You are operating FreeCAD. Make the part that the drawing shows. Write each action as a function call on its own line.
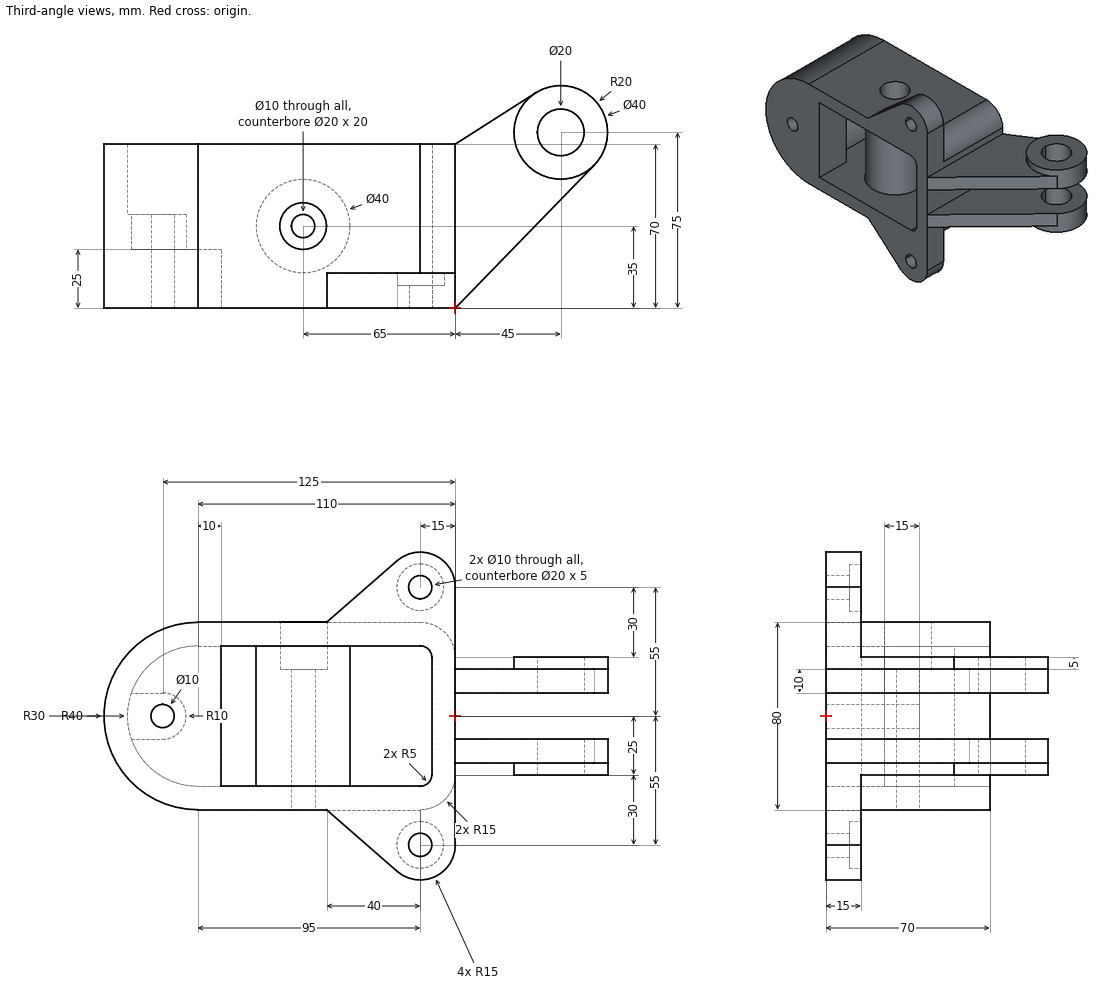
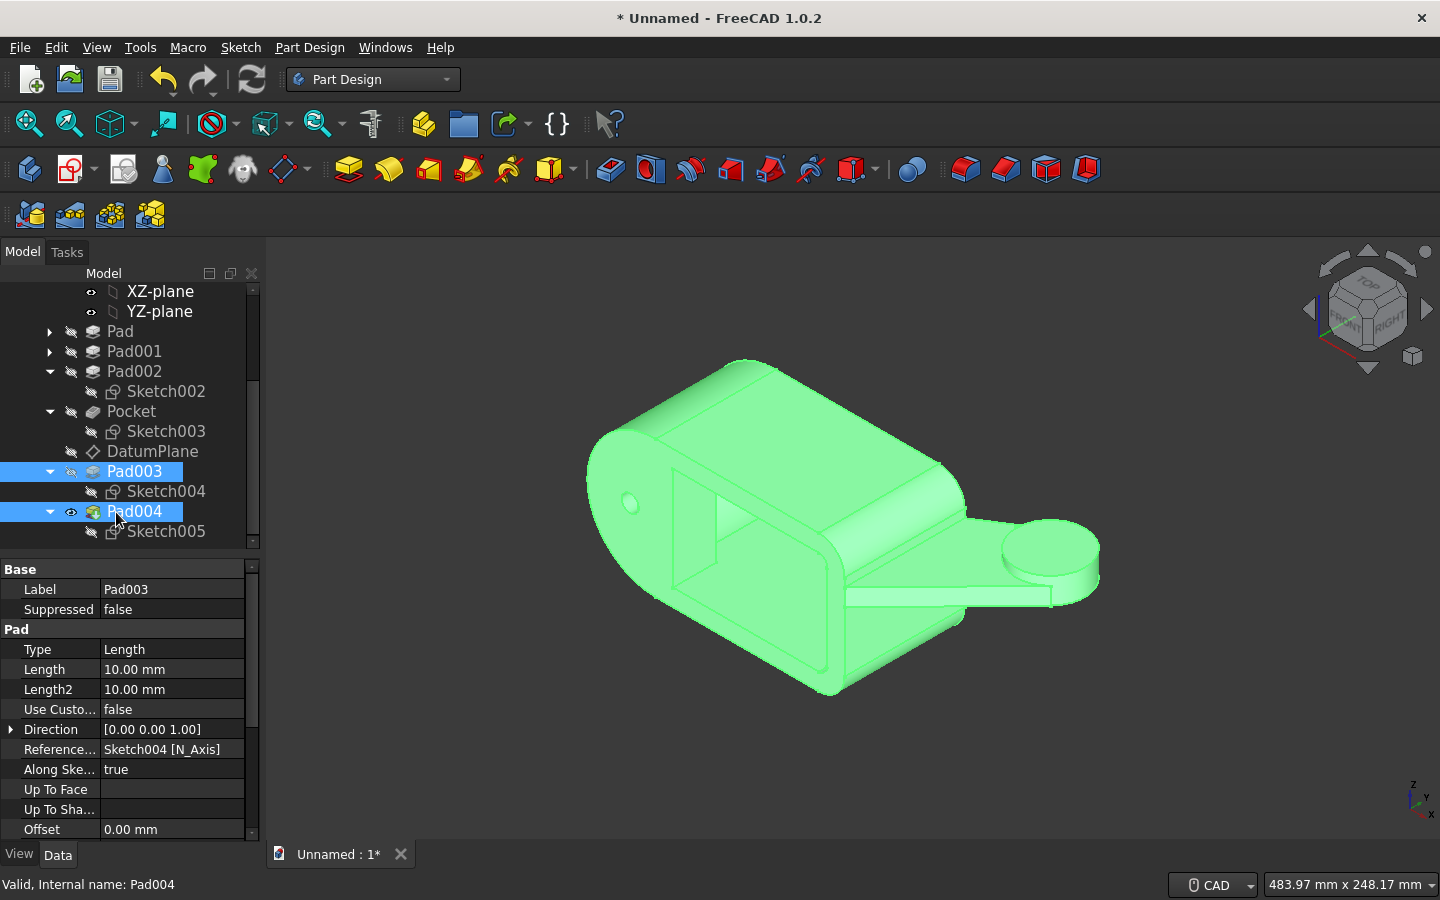
click(30, 214)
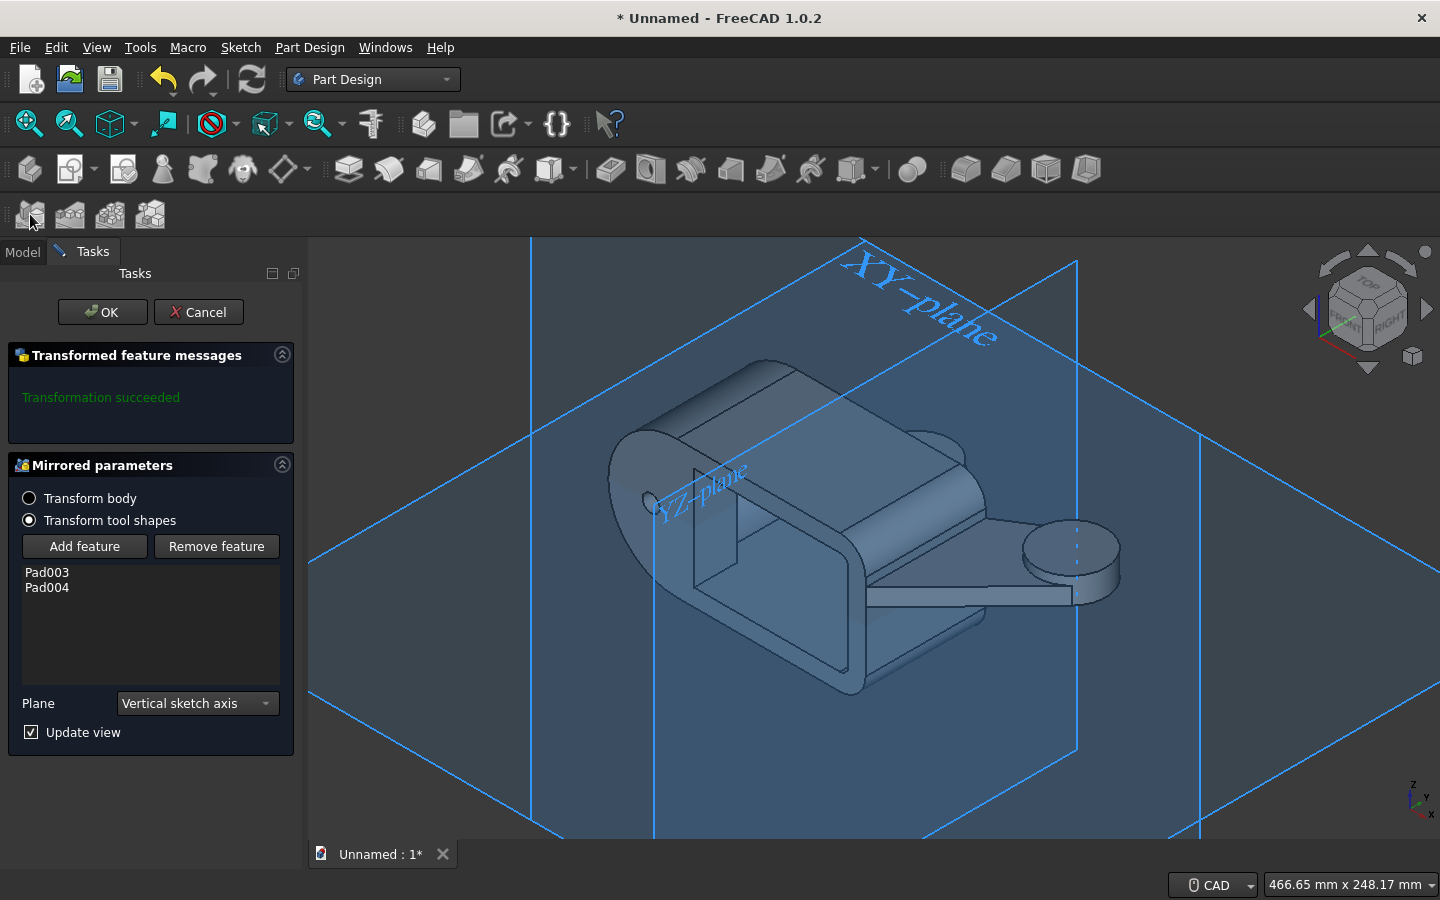
click(198, 704)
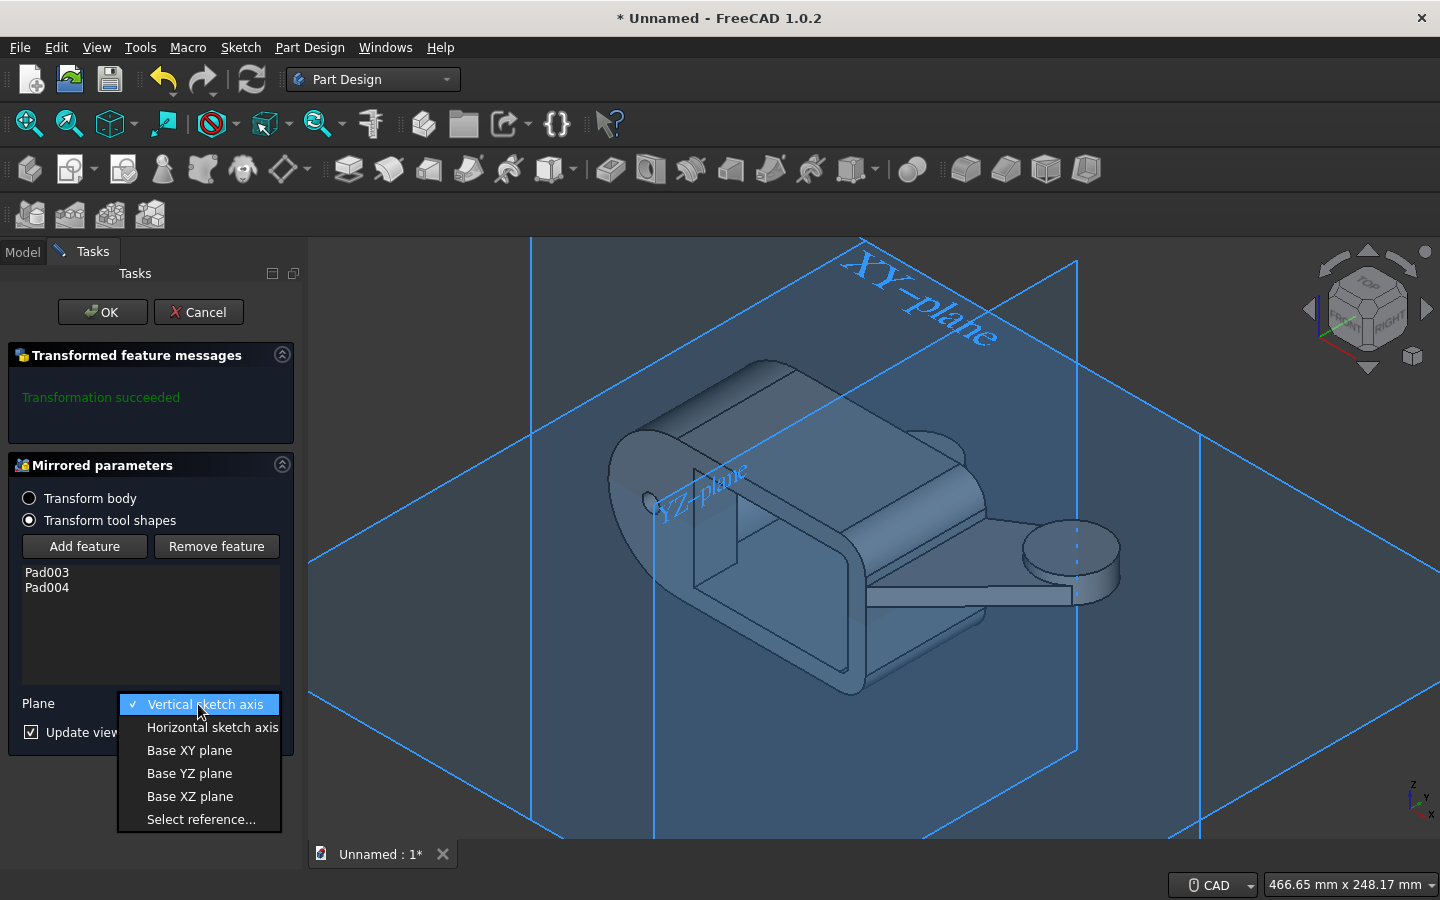
click(198, 750)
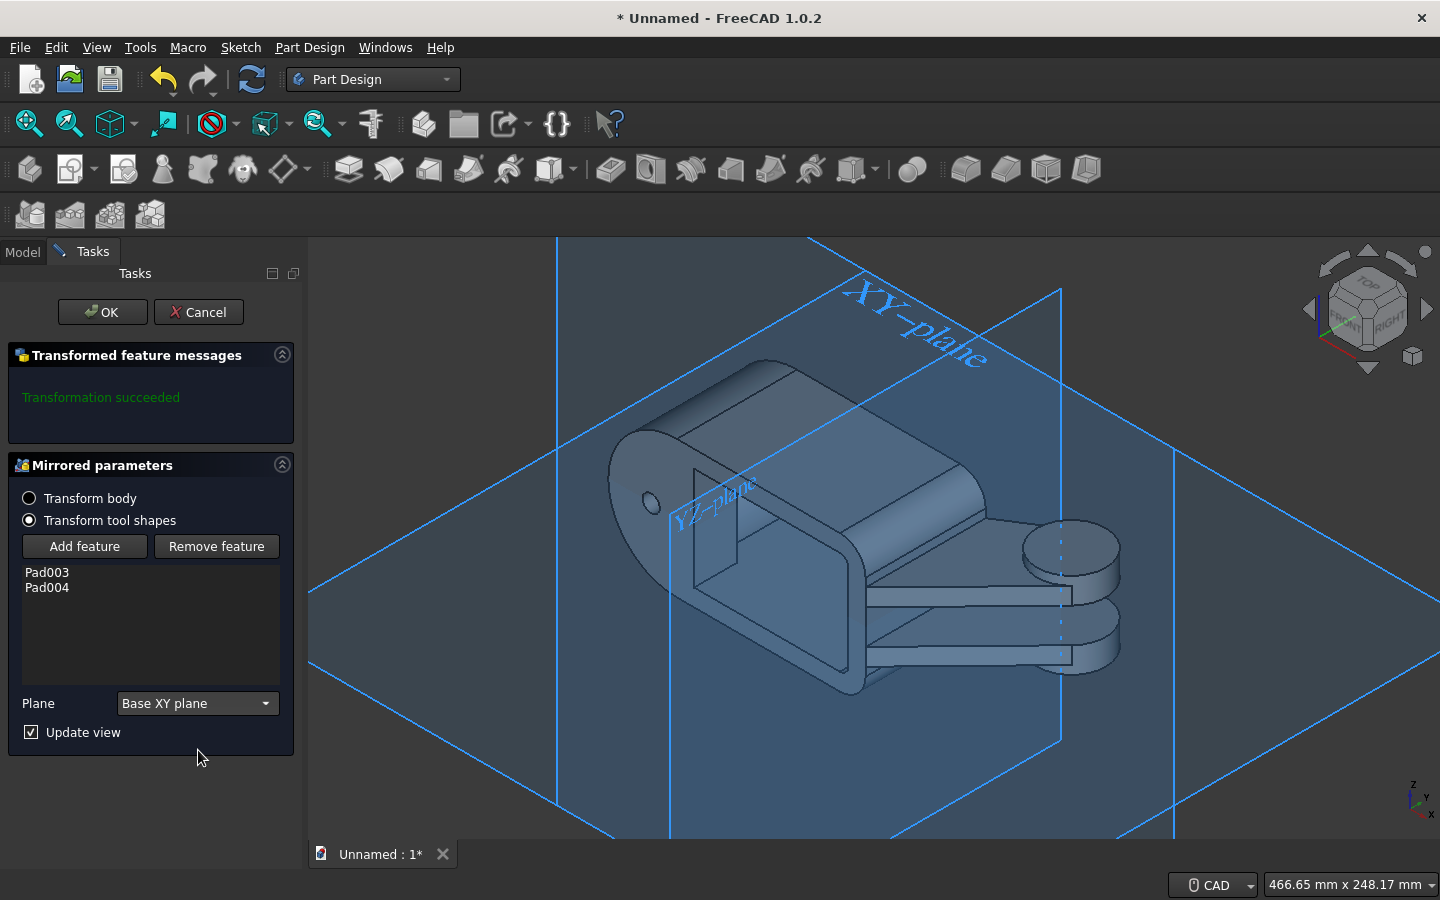
click(103, 312)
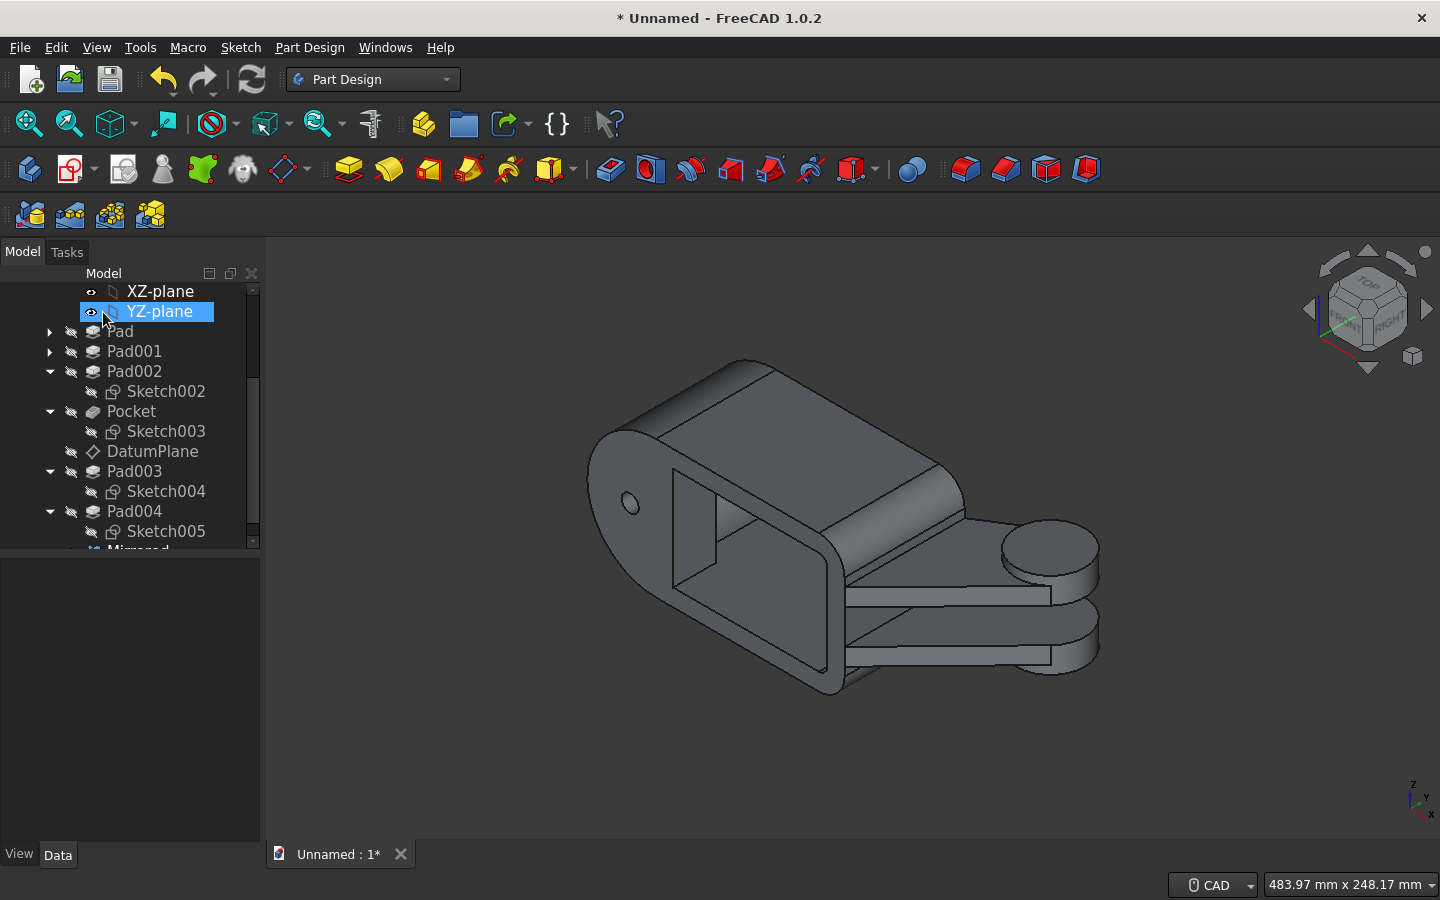
click(1050, 547)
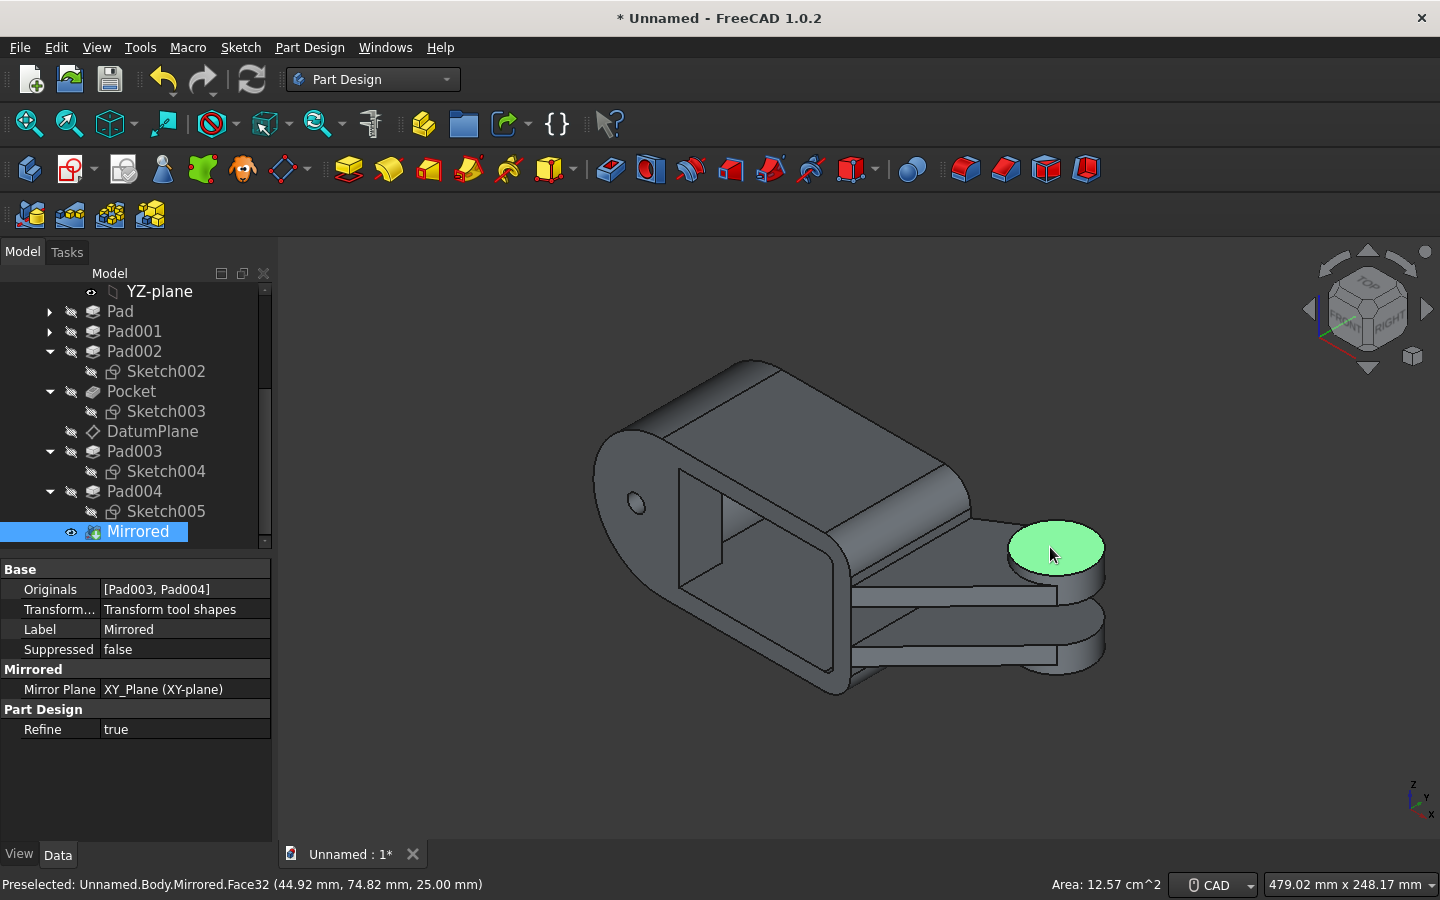
click(70, 170)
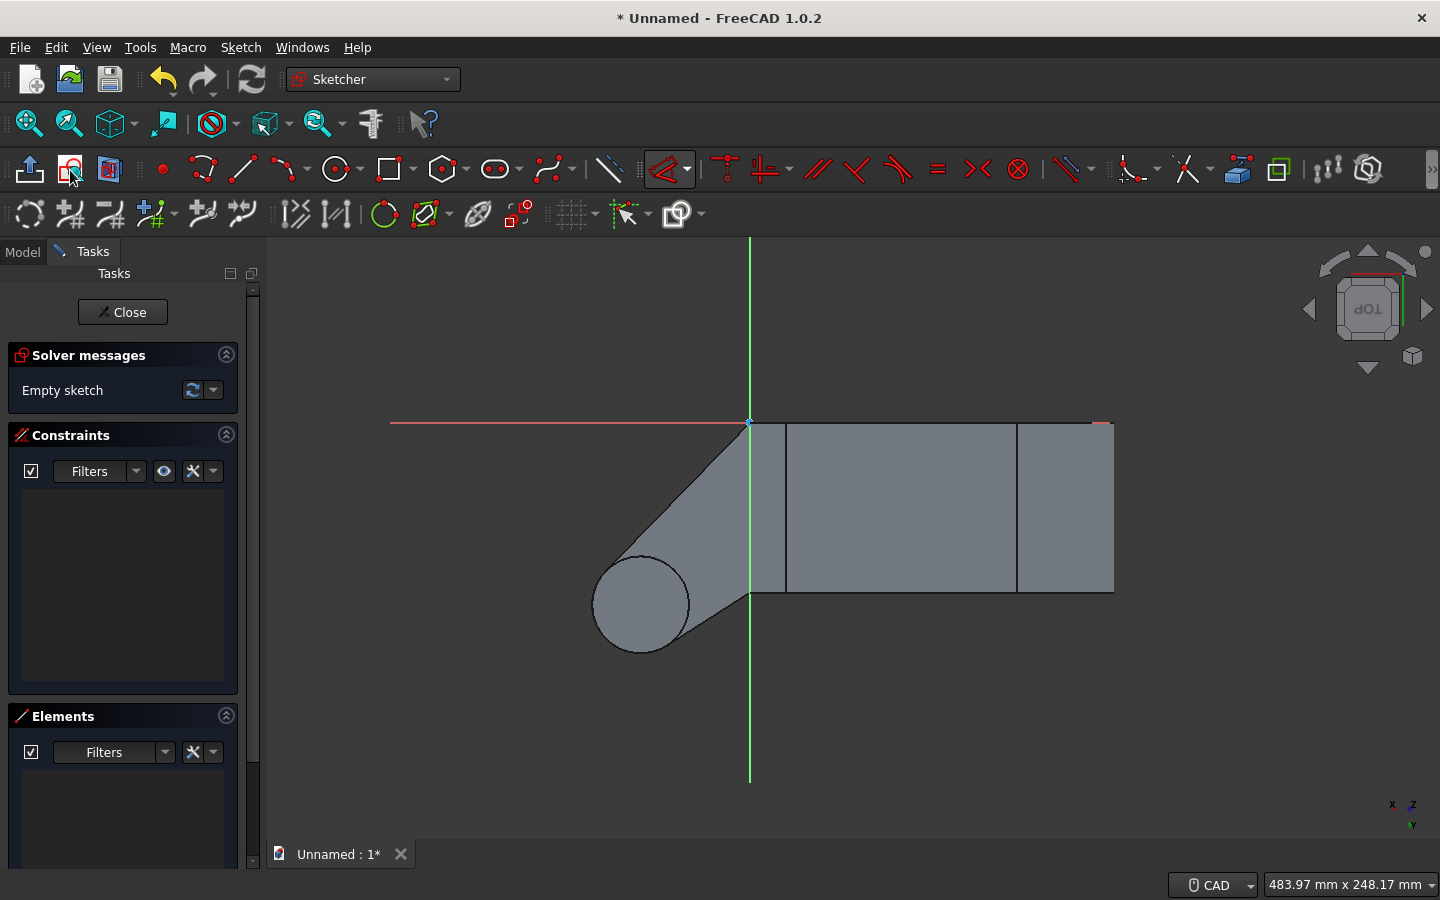
scroll(618, 615, up, 10)